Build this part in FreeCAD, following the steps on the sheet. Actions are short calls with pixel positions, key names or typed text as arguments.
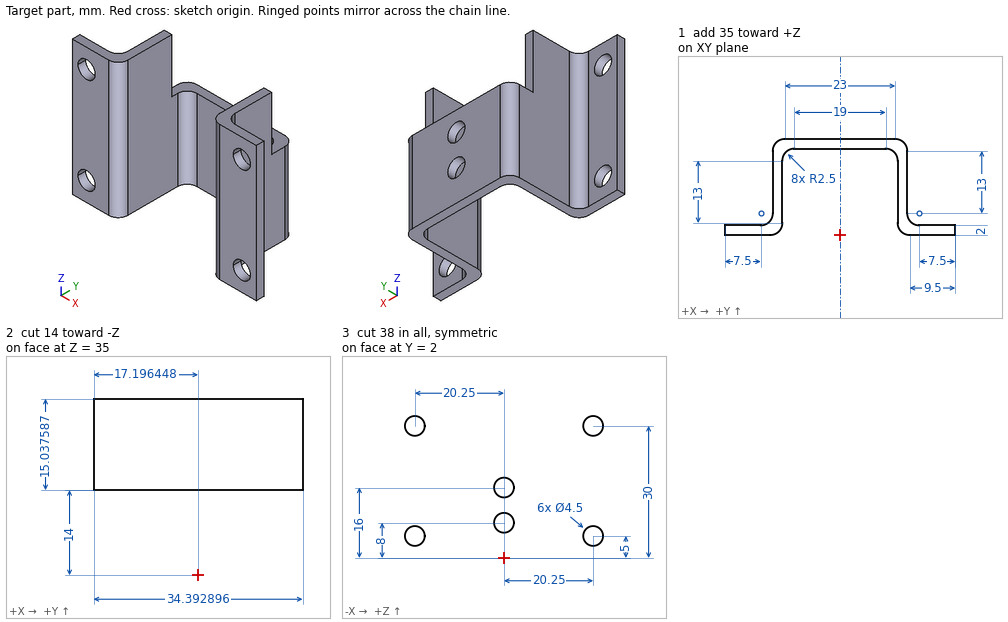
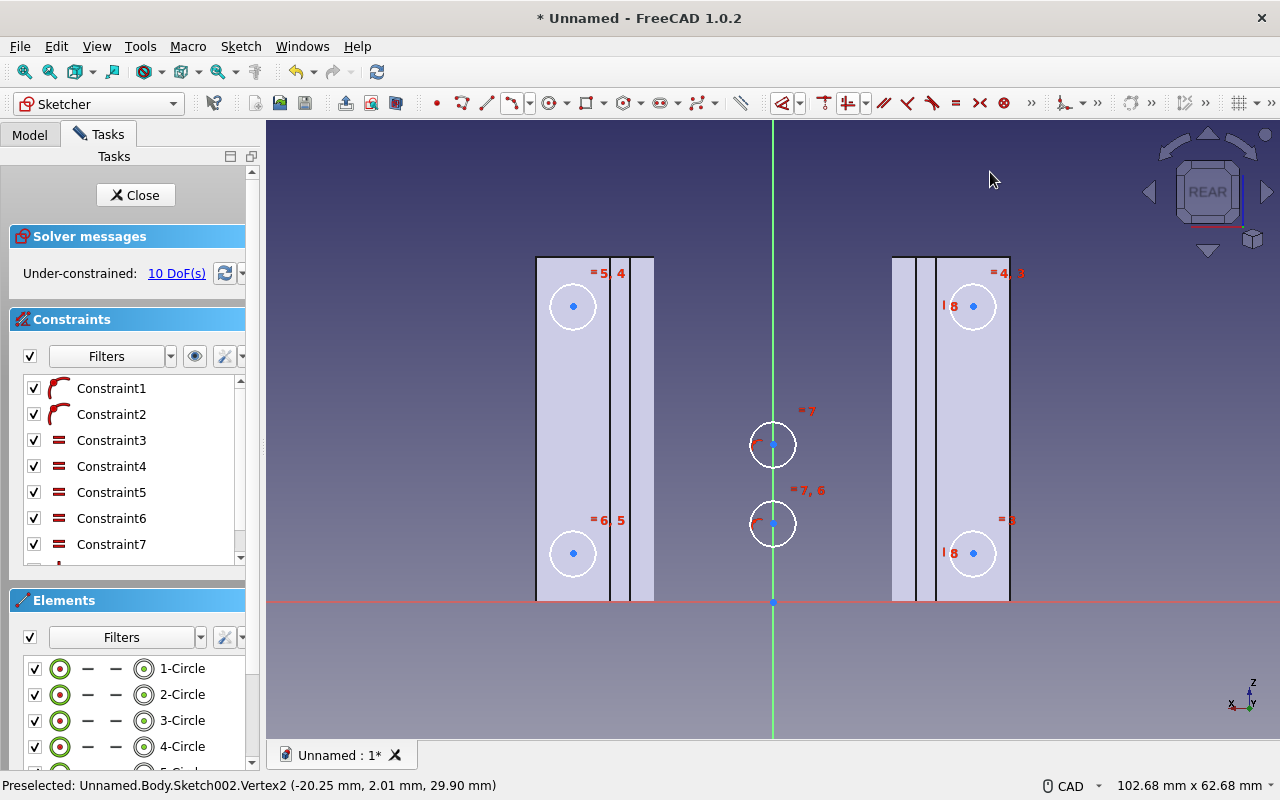
click(973, 307)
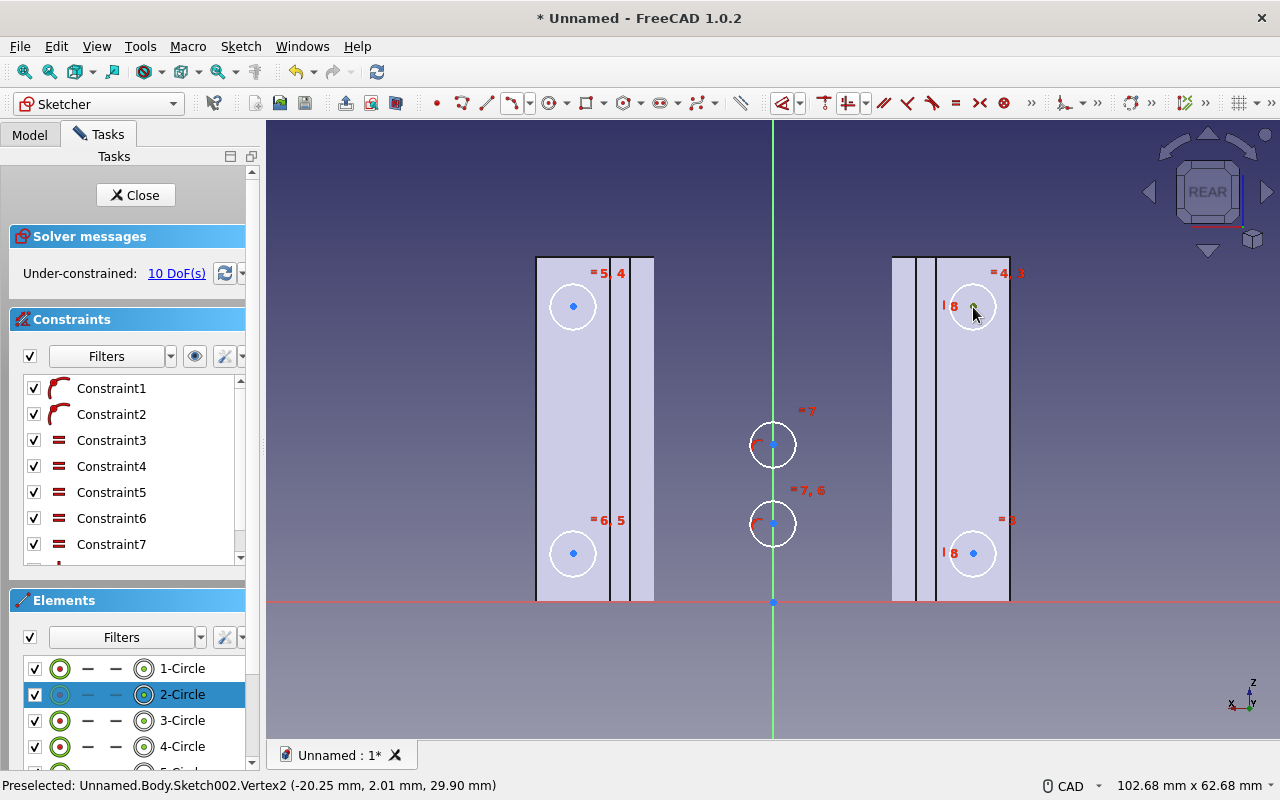
click(573, 307)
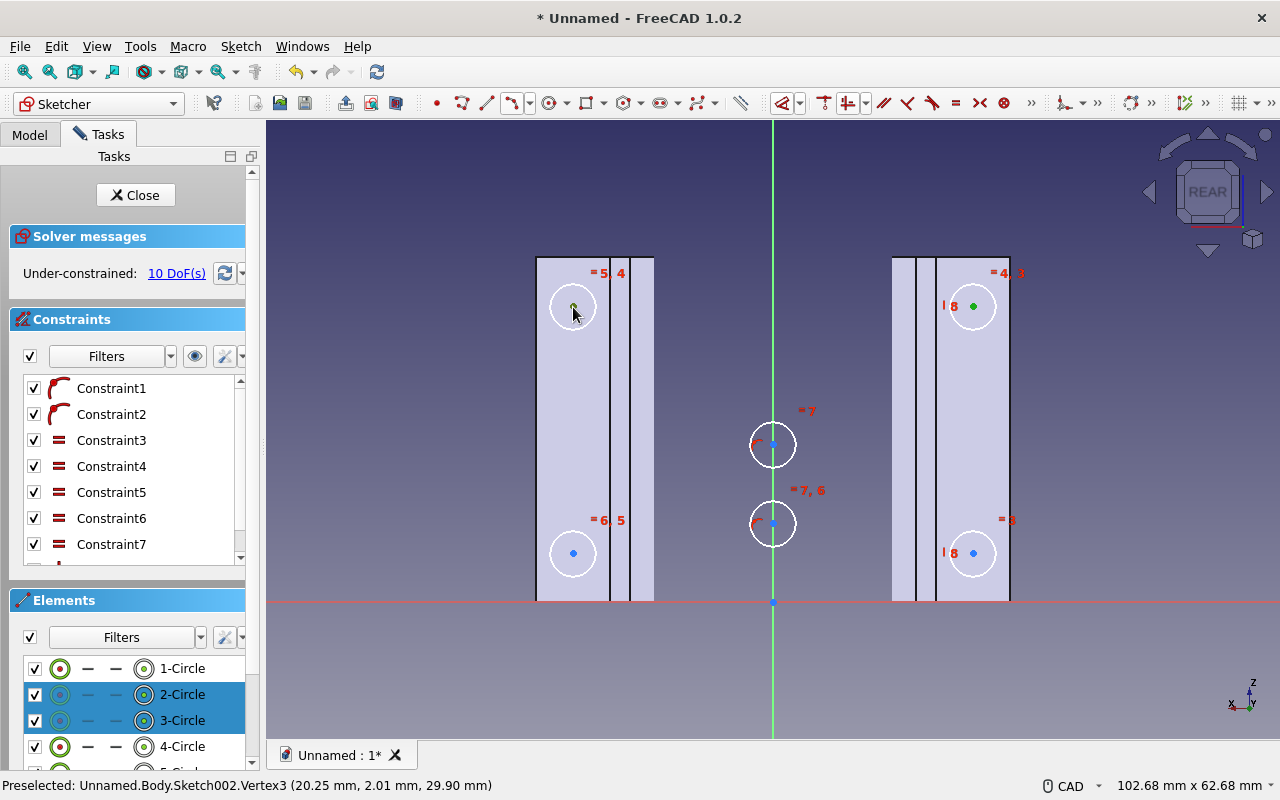
click(866, 104)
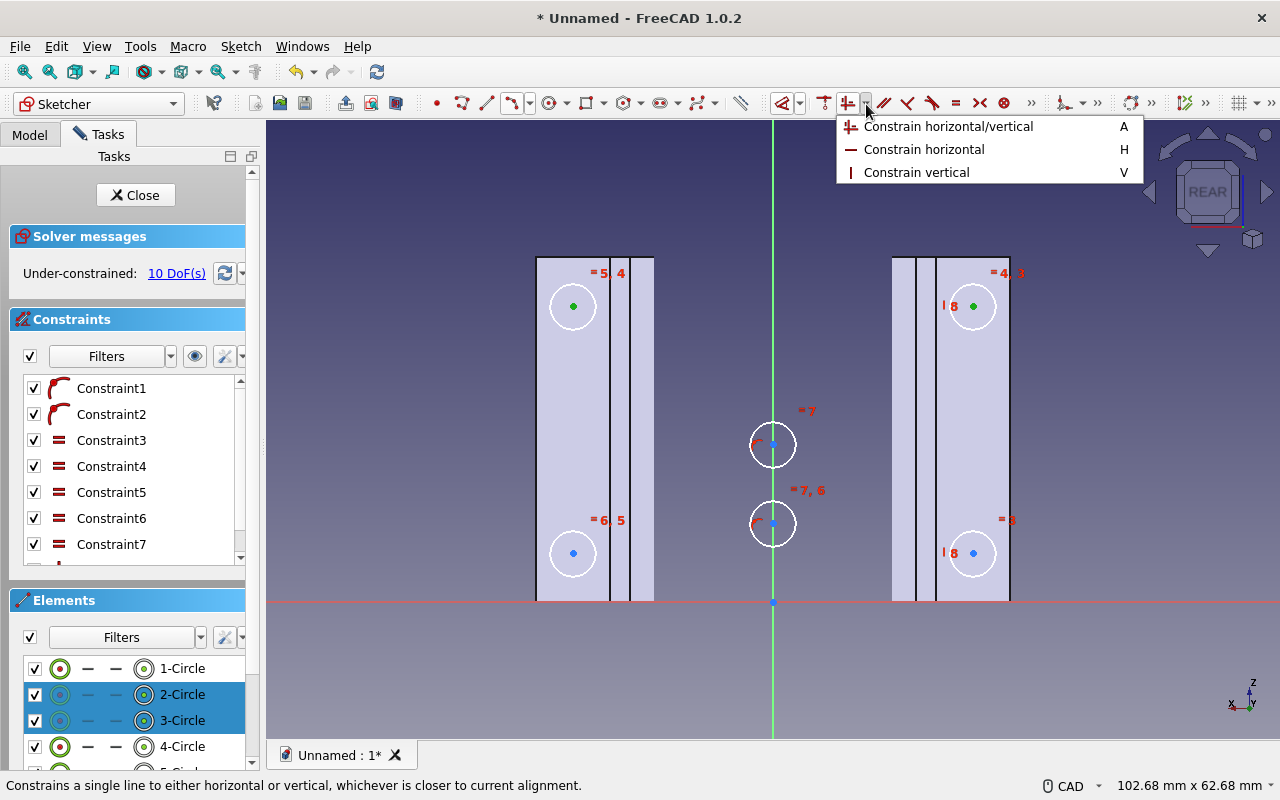
click(990, 150)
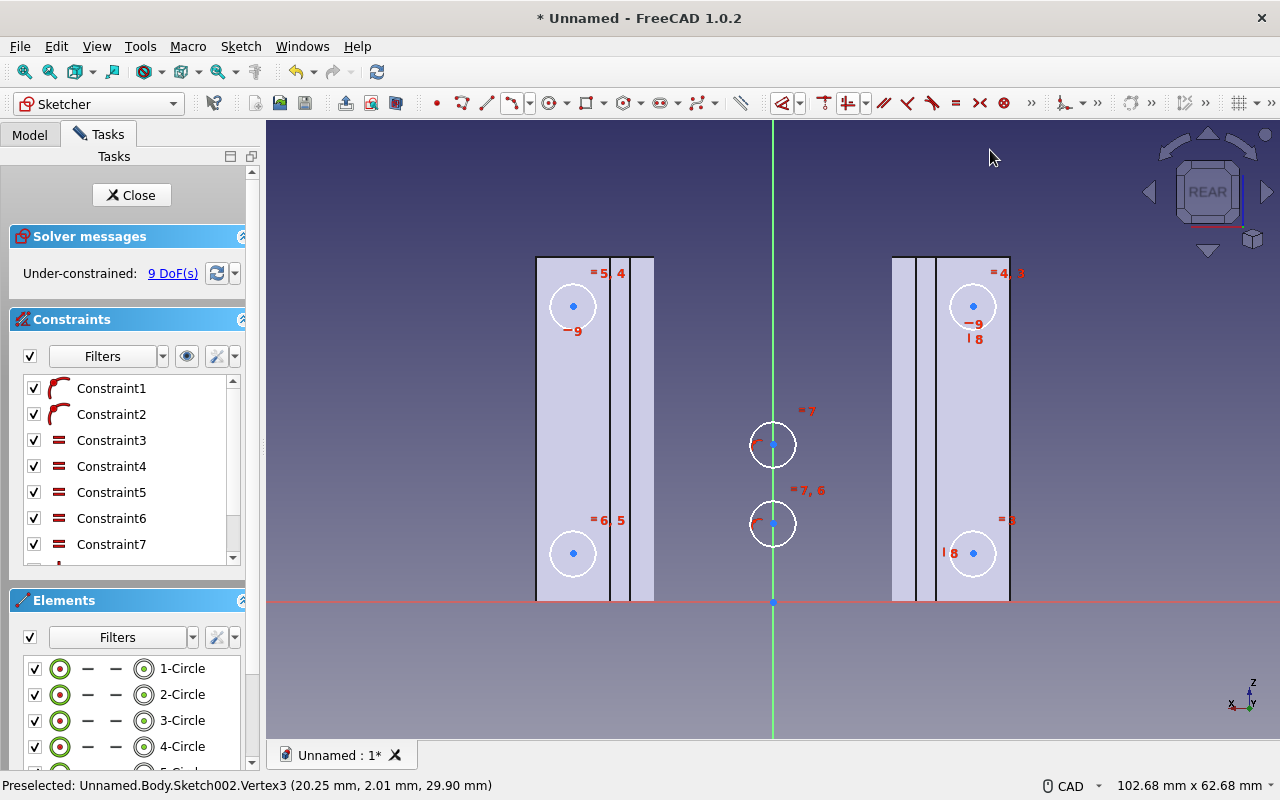
click(573, 307)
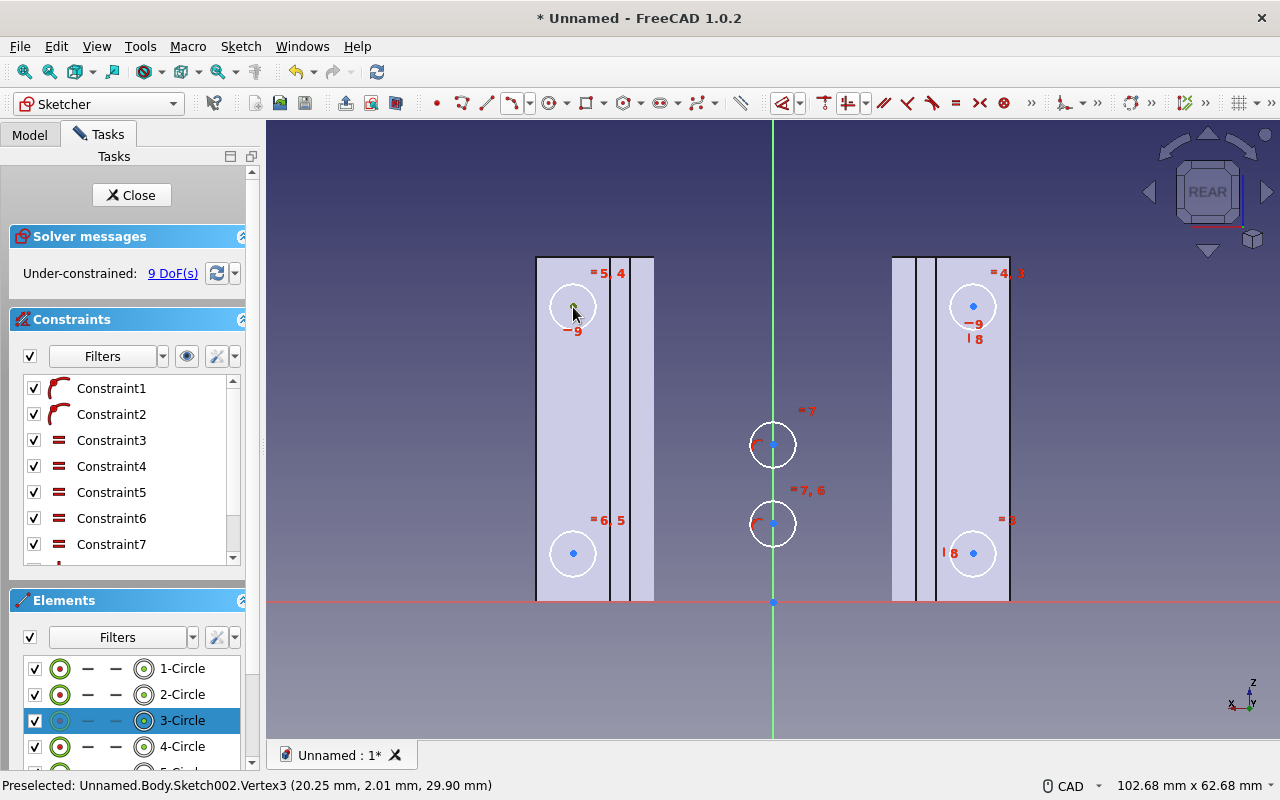
click(573, 554)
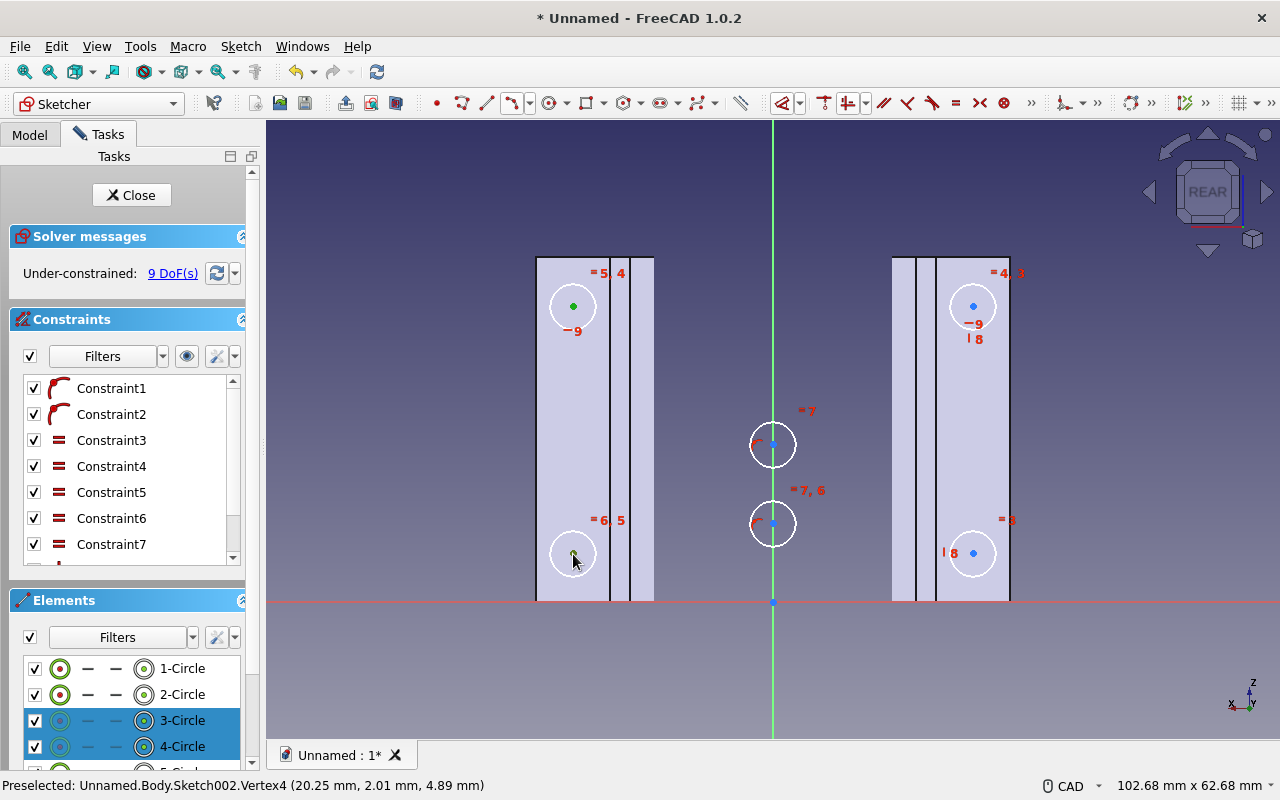
click(866, 104)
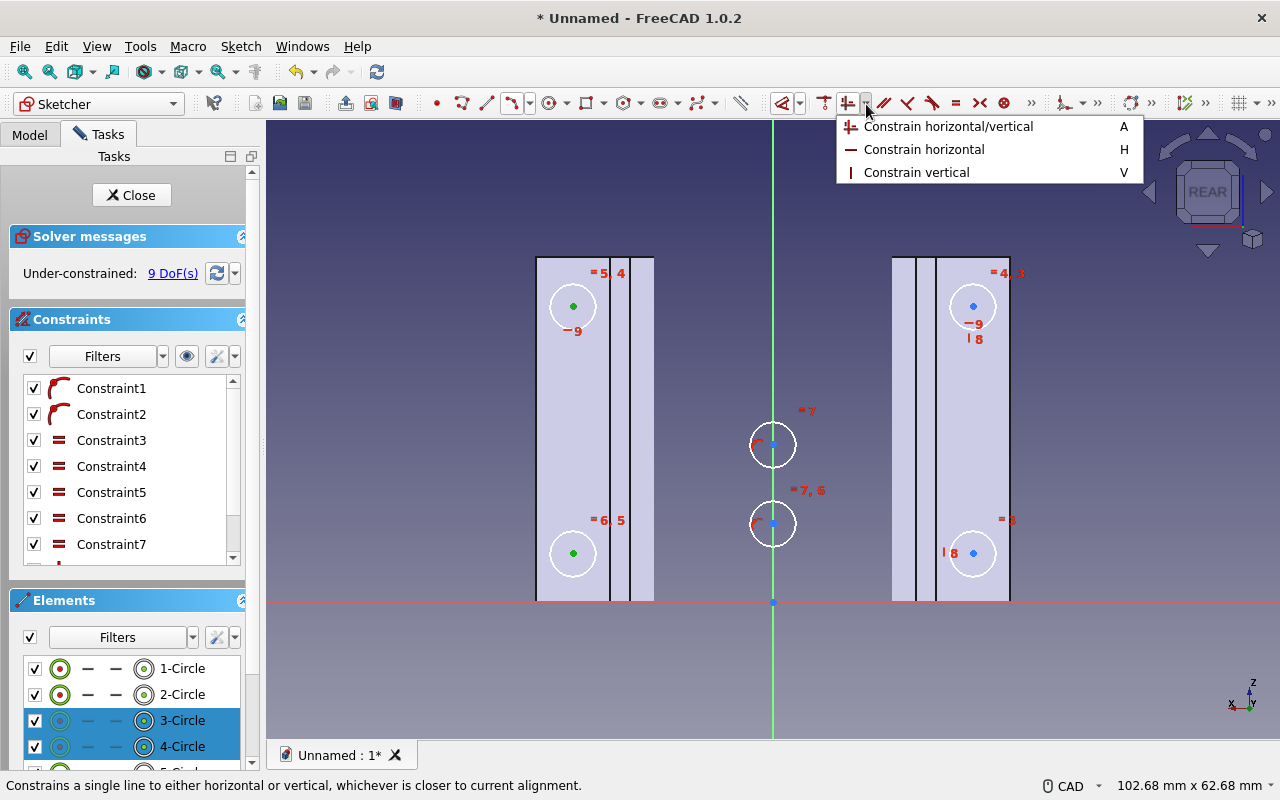
click(990, 172)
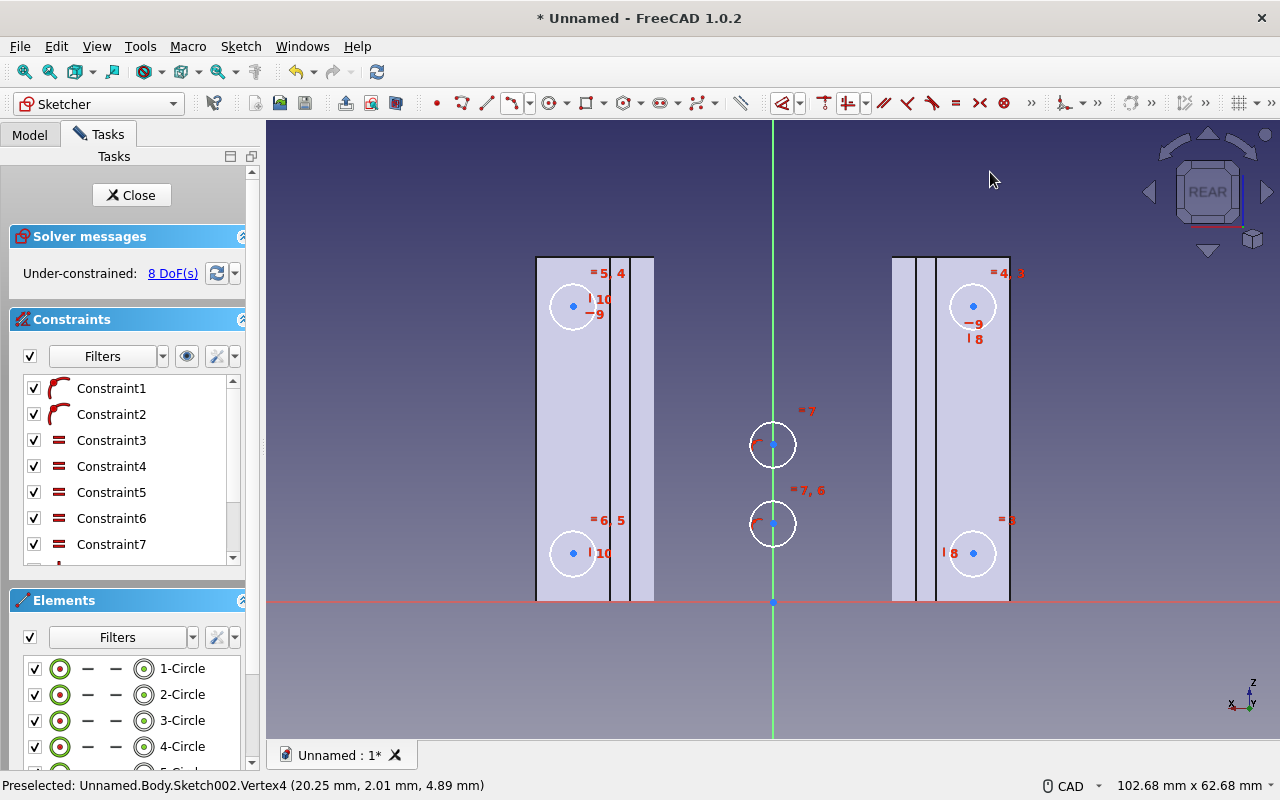
click(973, 554)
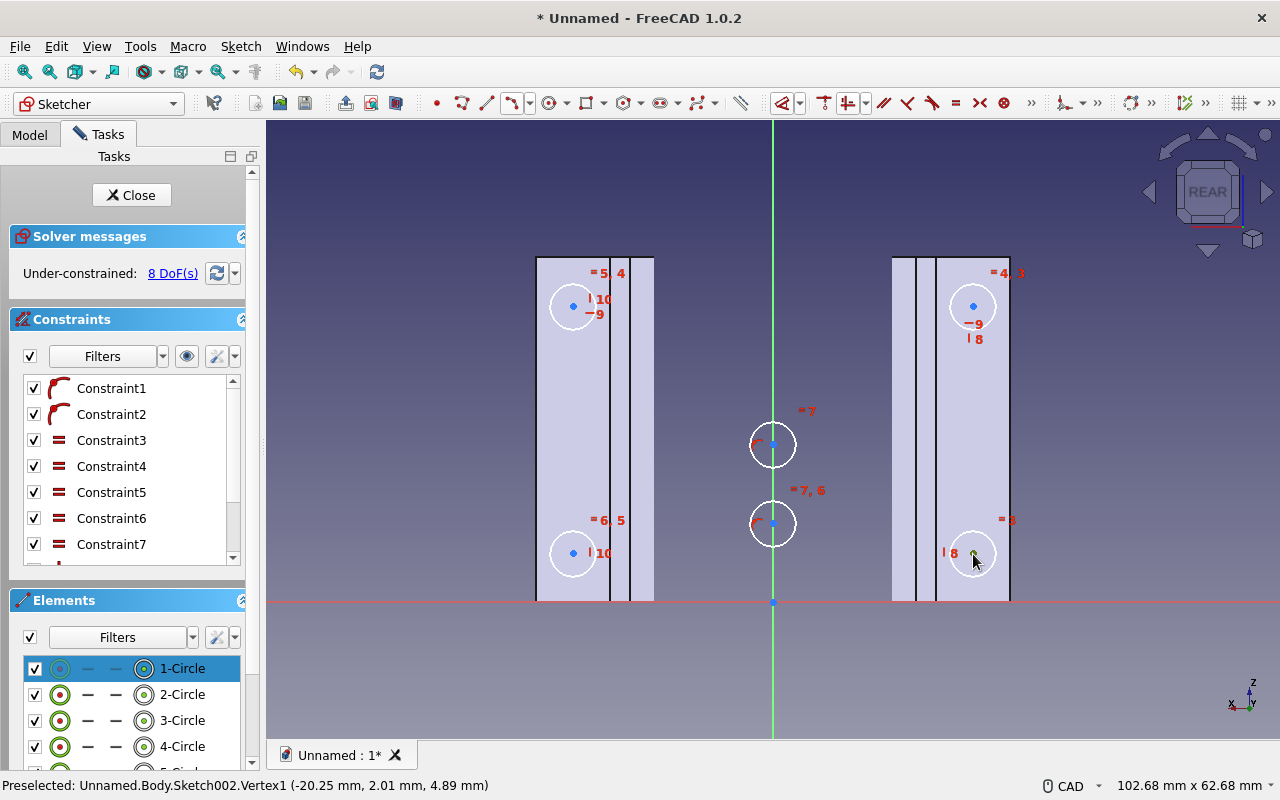
click(573, 554)